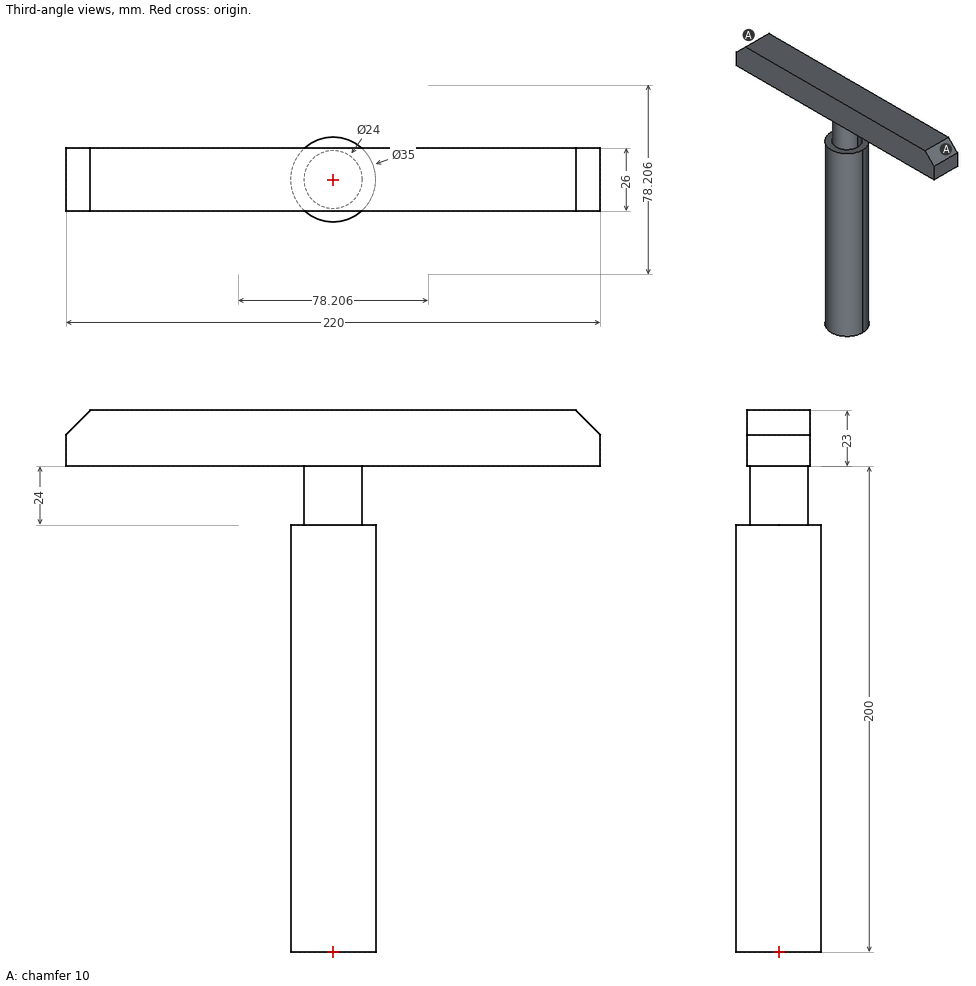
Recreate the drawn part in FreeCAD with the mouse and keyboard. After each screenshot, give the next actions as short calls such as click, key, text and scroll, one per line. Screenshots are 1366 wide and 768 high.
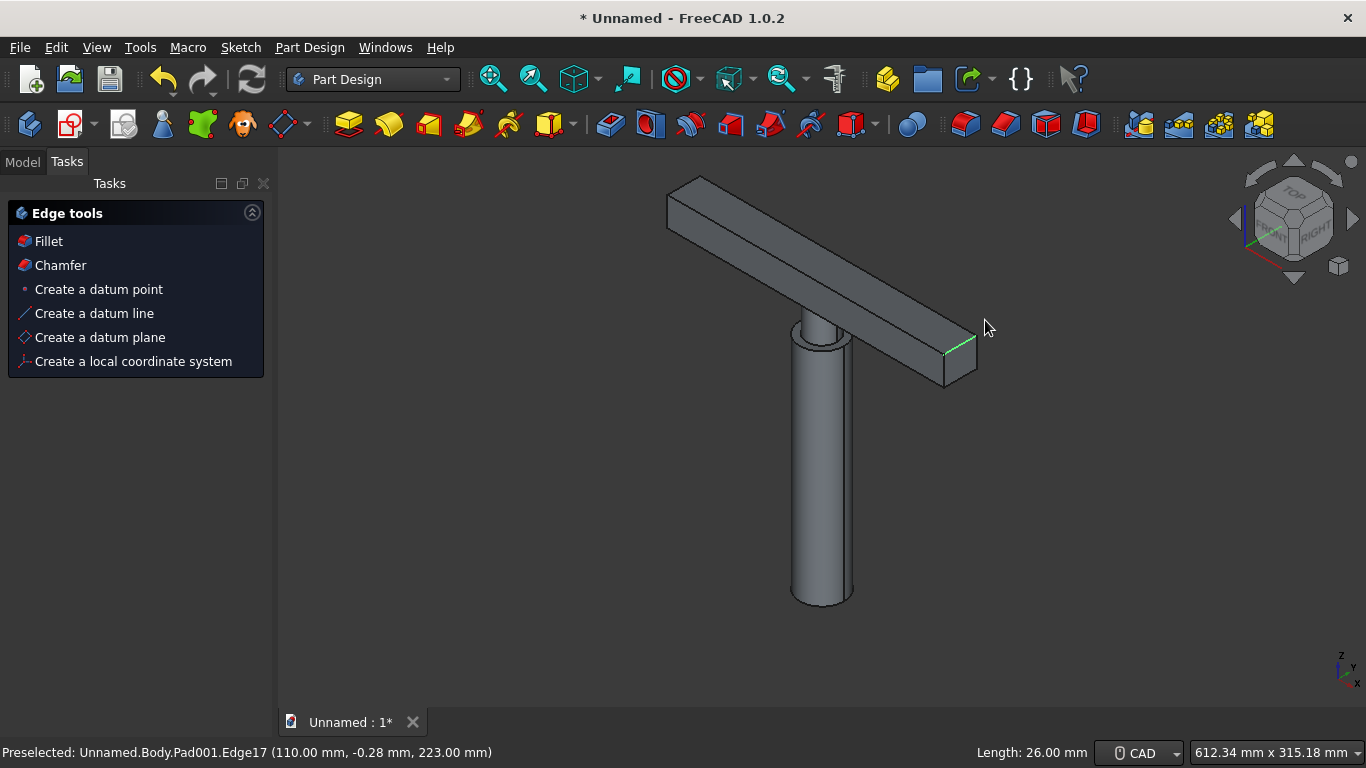
key(2)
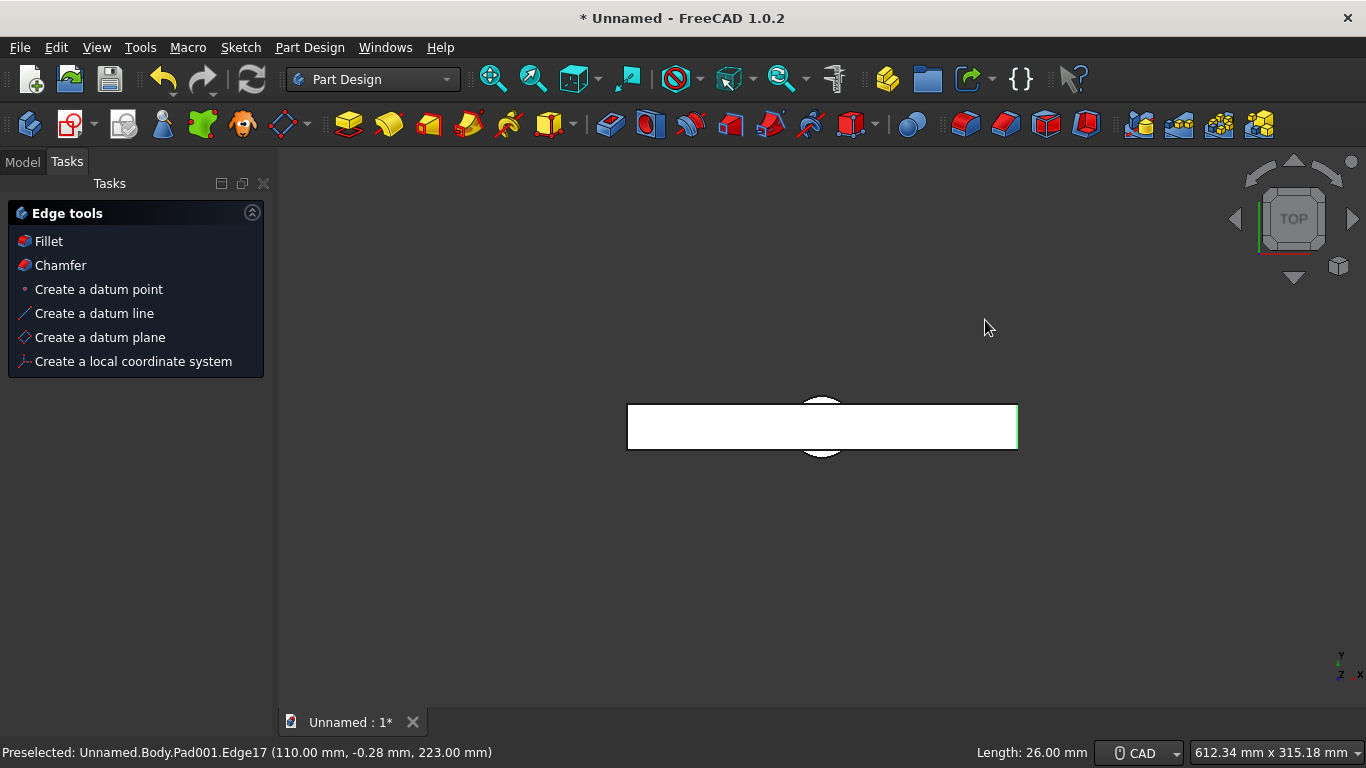
key(v)
key(f)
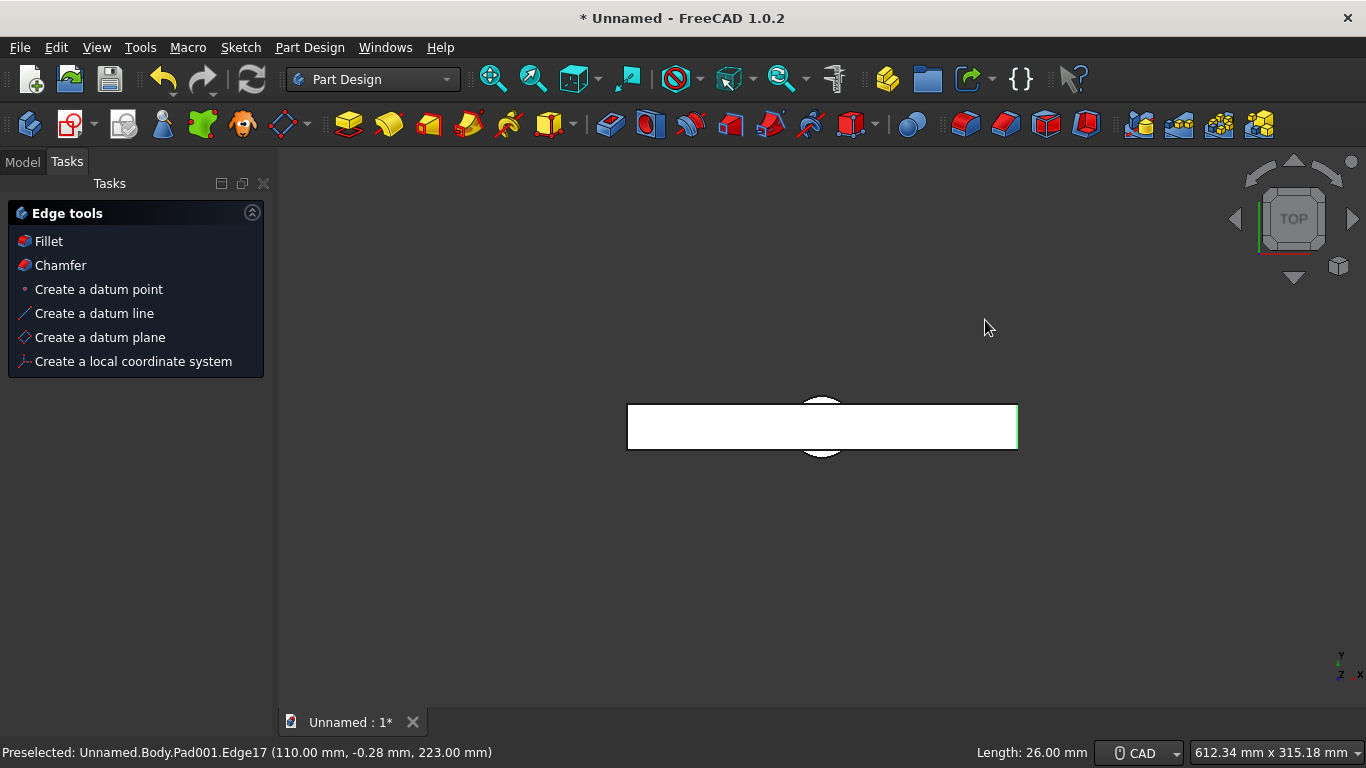
click(627, 426, ctrl)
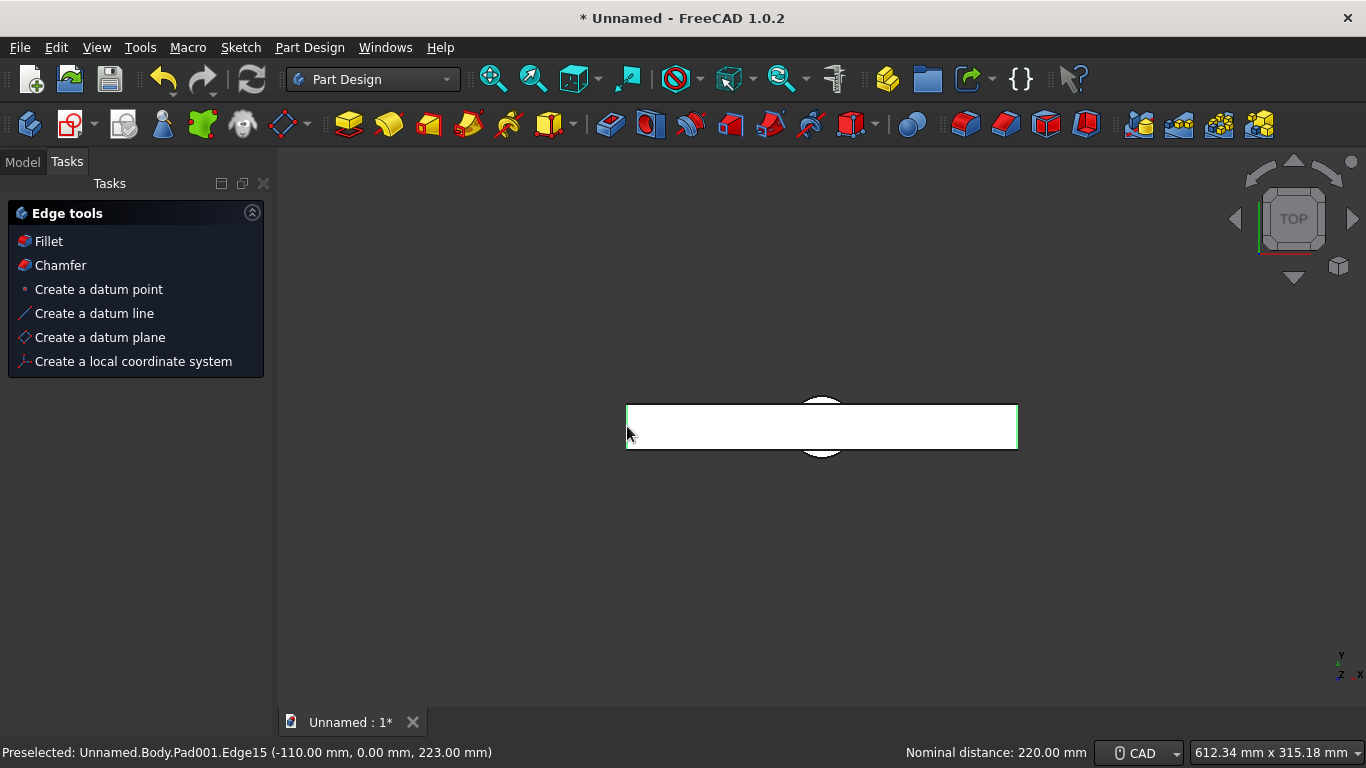
click(1006, 124)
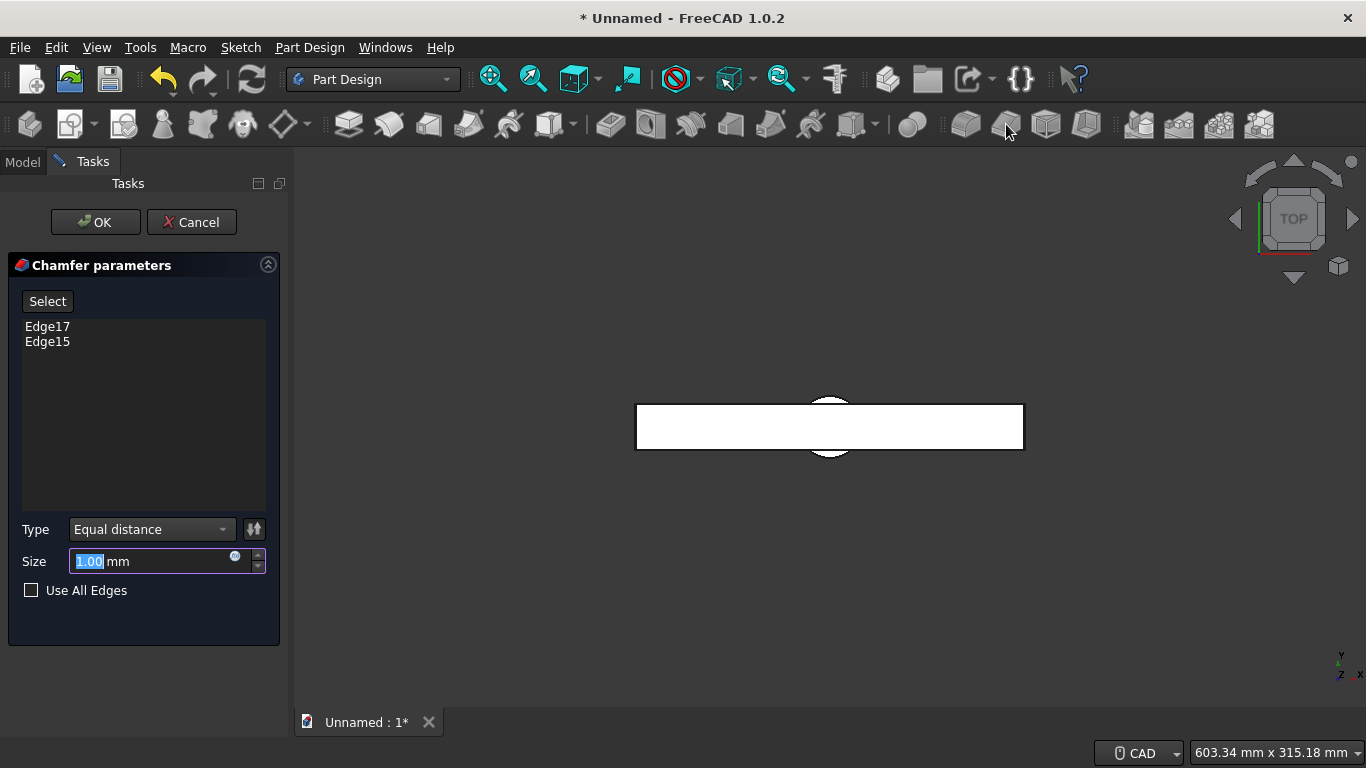
text(10)
key(Tab)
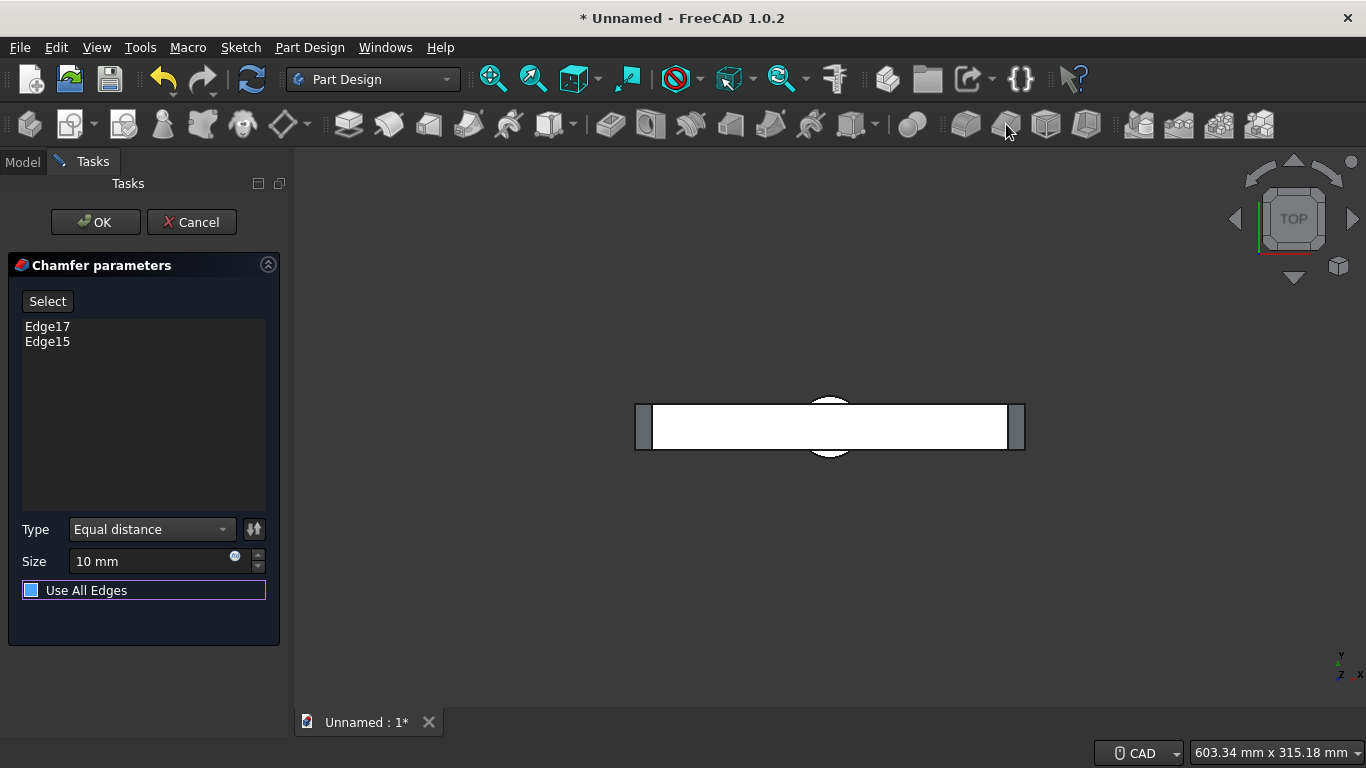
click(96, 222)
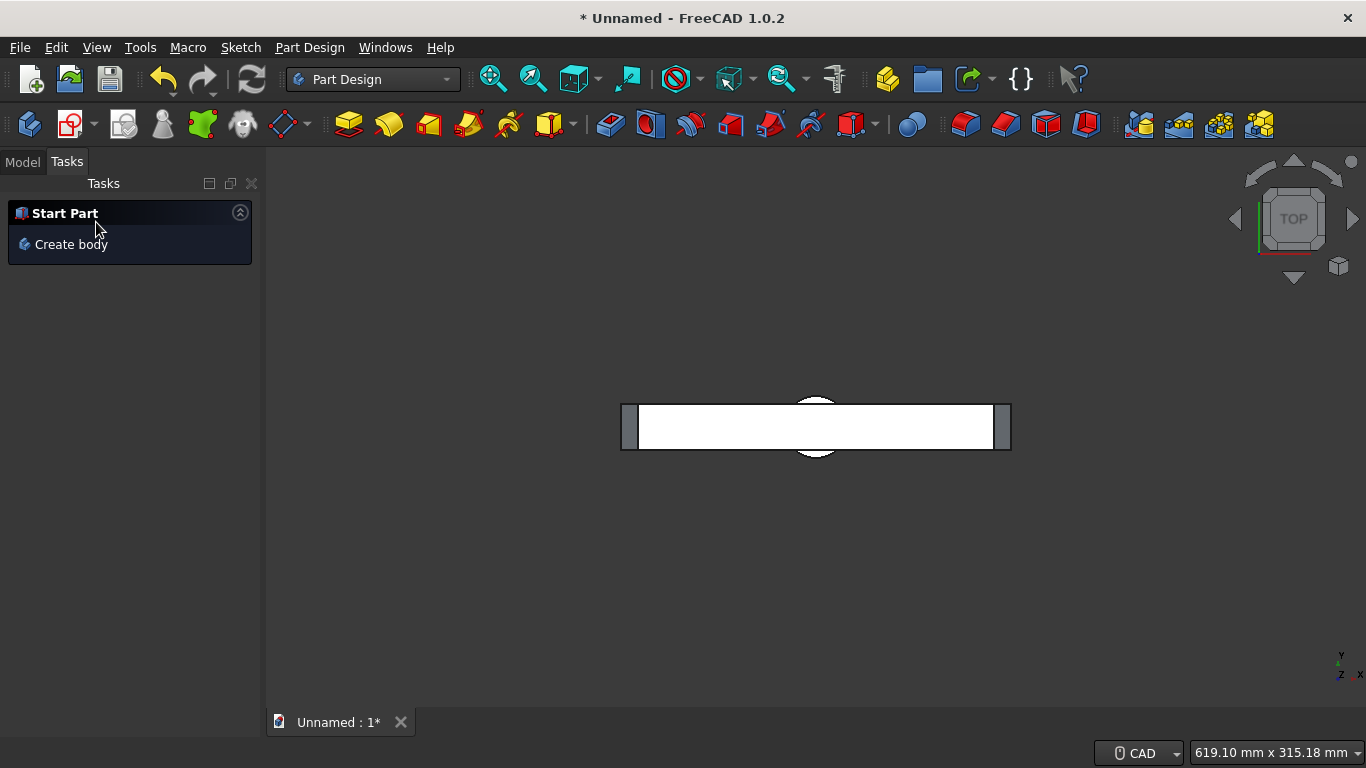
key(0)